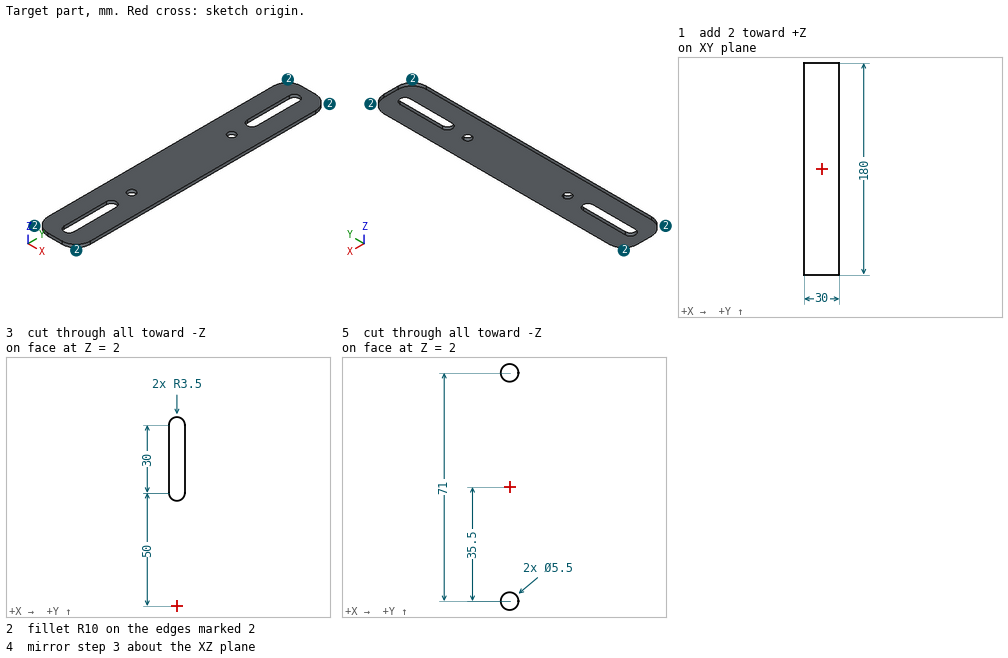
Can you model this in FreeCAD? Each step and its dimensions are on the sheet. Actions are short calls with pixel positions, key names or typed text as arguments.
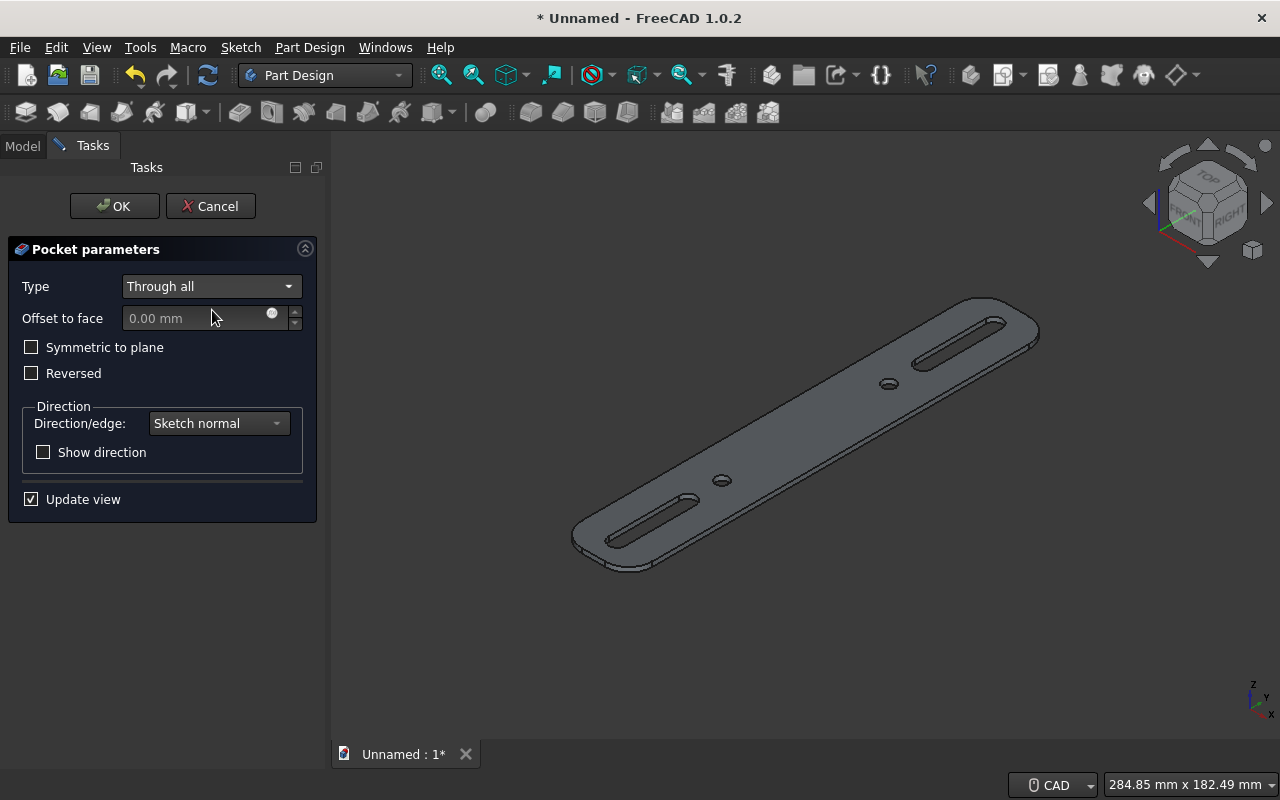
click(115, 206)